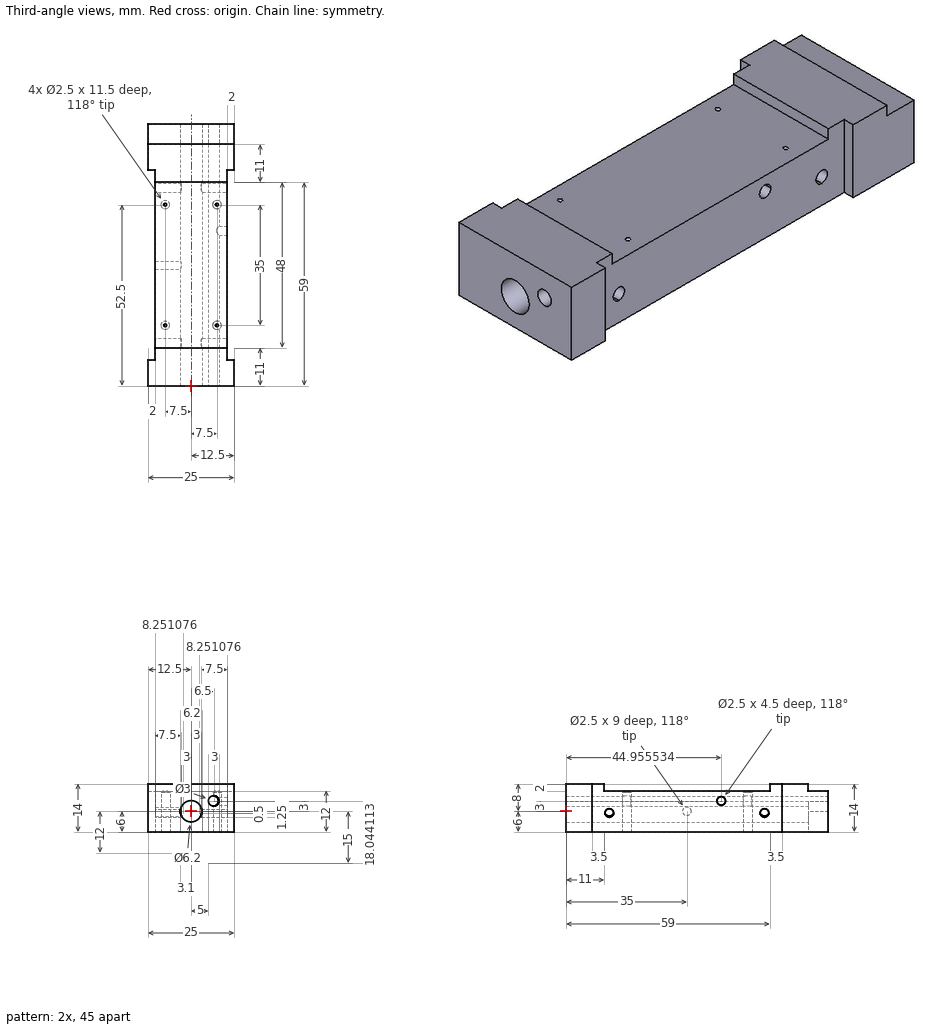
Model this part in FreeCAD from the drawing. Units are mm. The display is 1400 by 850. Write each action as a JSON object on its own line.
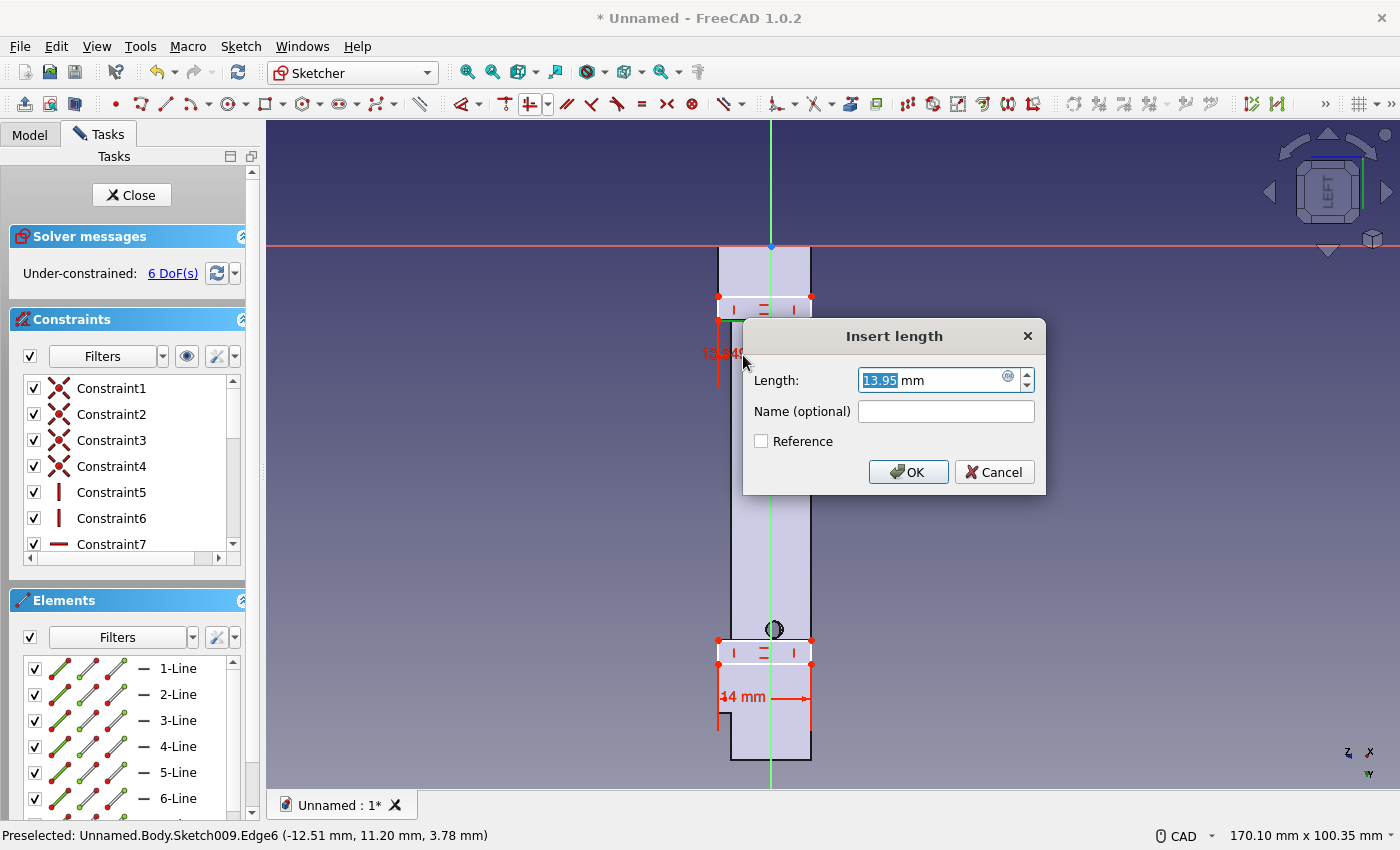
{"action": "type", "text": "14"}
{"action": "key", "text": "Return"}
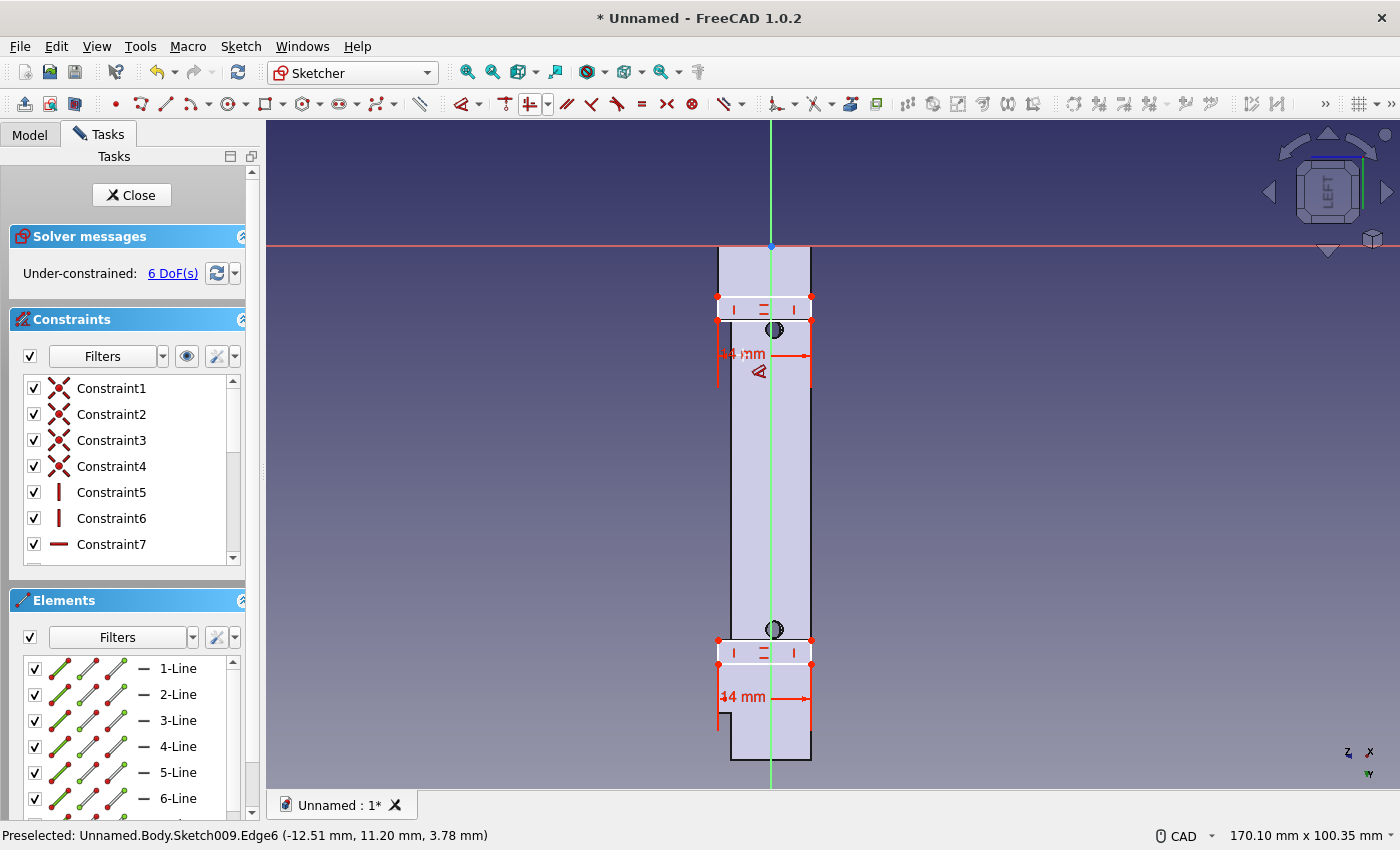
{"action": "left_click", "coordinate": [718, 641]}
{"action": "left_click", "coordinate": [745, 212]}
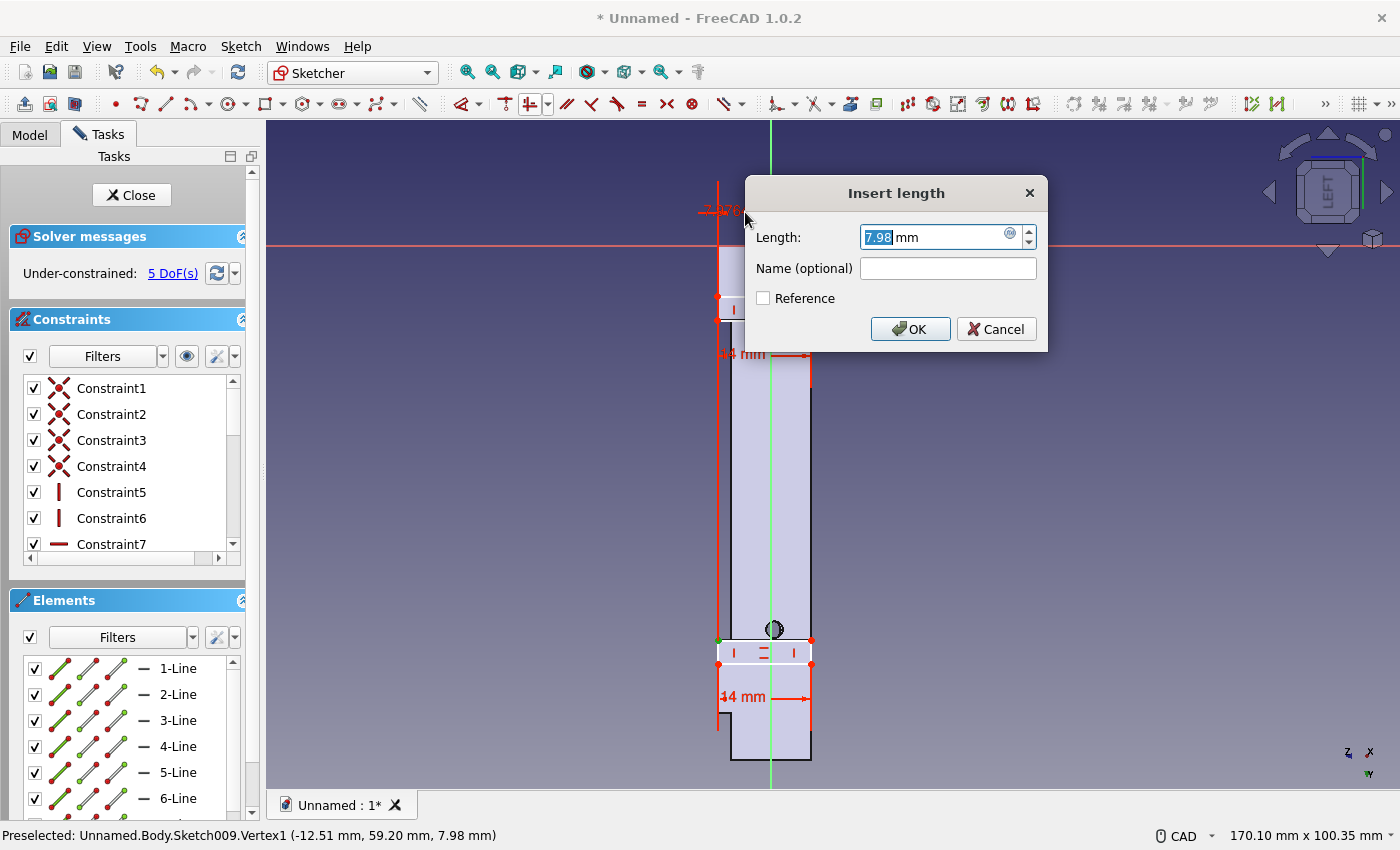
{"action": "type", "text": "8"}
{"action": "key", "text": "Return"}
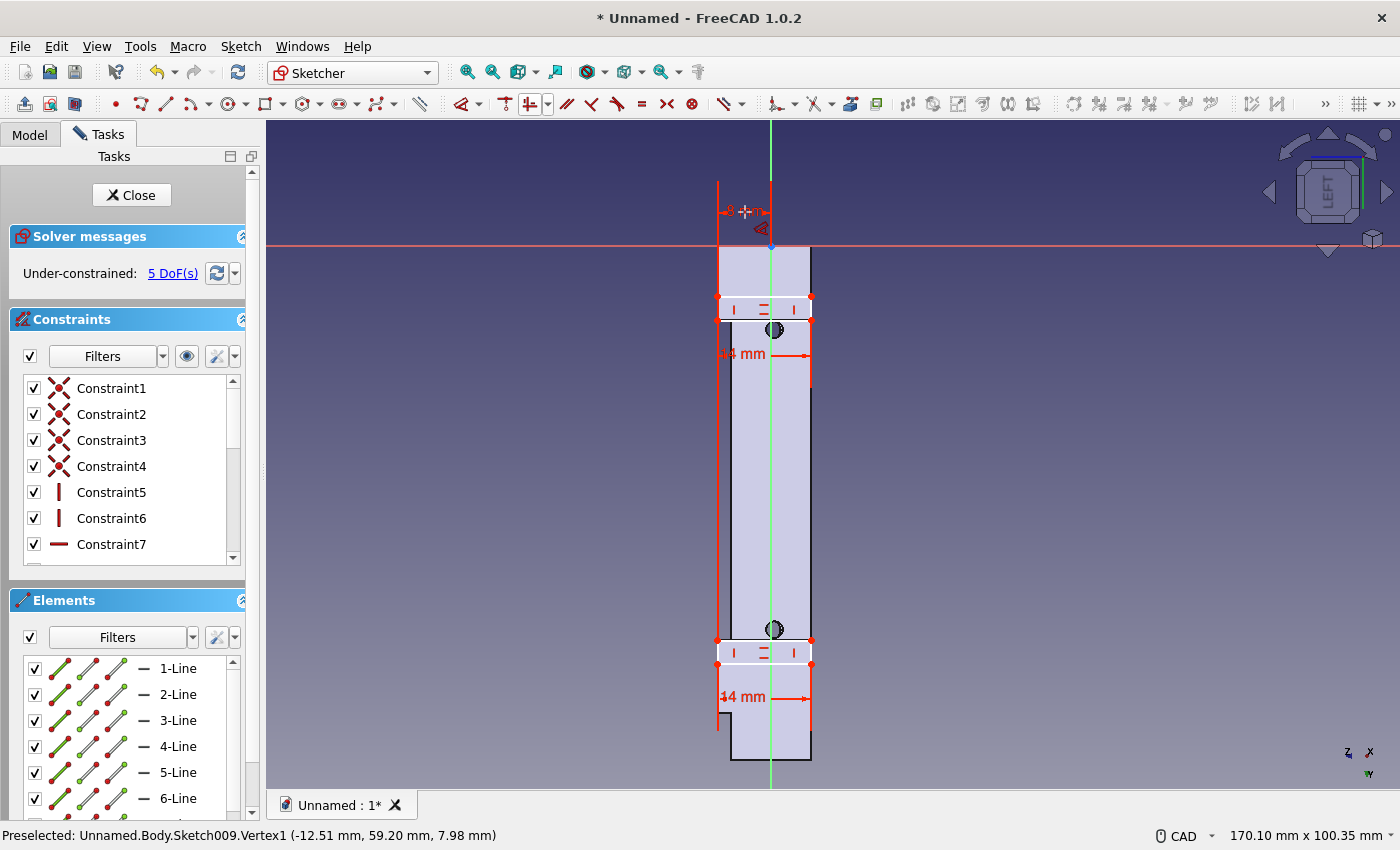
{"action": "left_click", "coordinate": [718, 297]}
{"action": "left_click", "coordinate": [744, 188]}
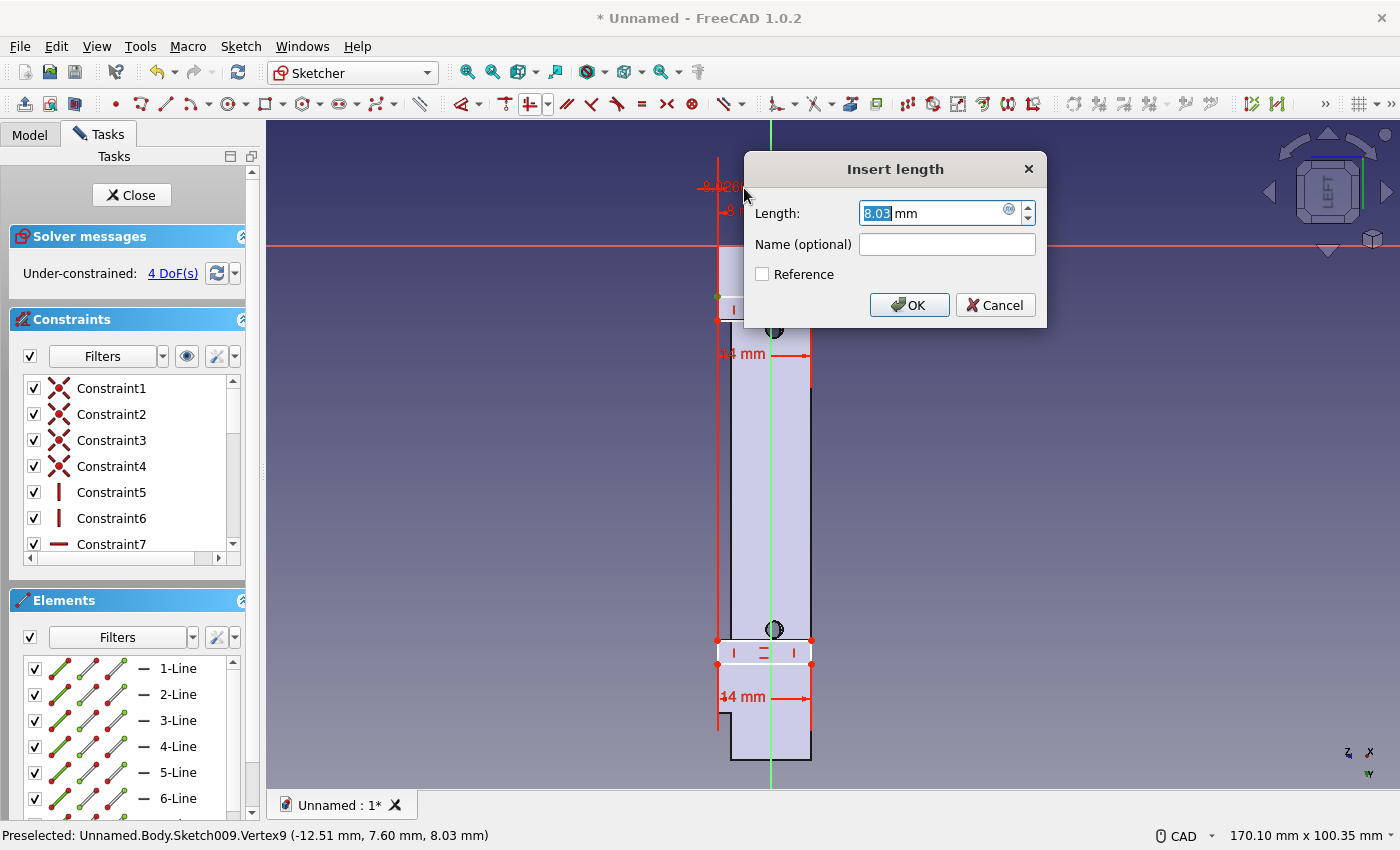
{"action": "type", "text": "8"}
{"action": "key", "text": "Return"}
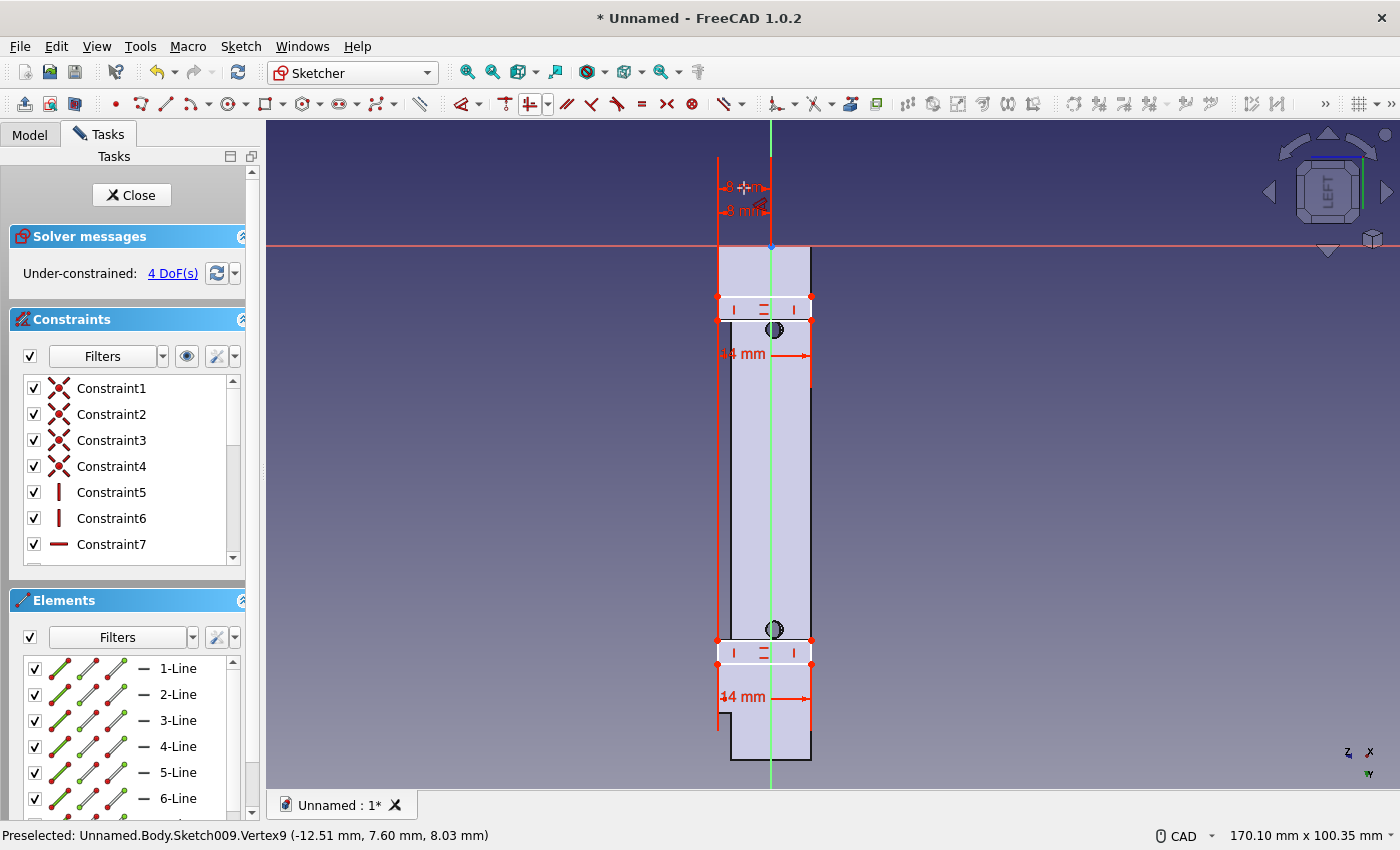
{"action": "scroll", "coordinate": [718, 650], "scroll_direction": "up", "scroll_amount": 3}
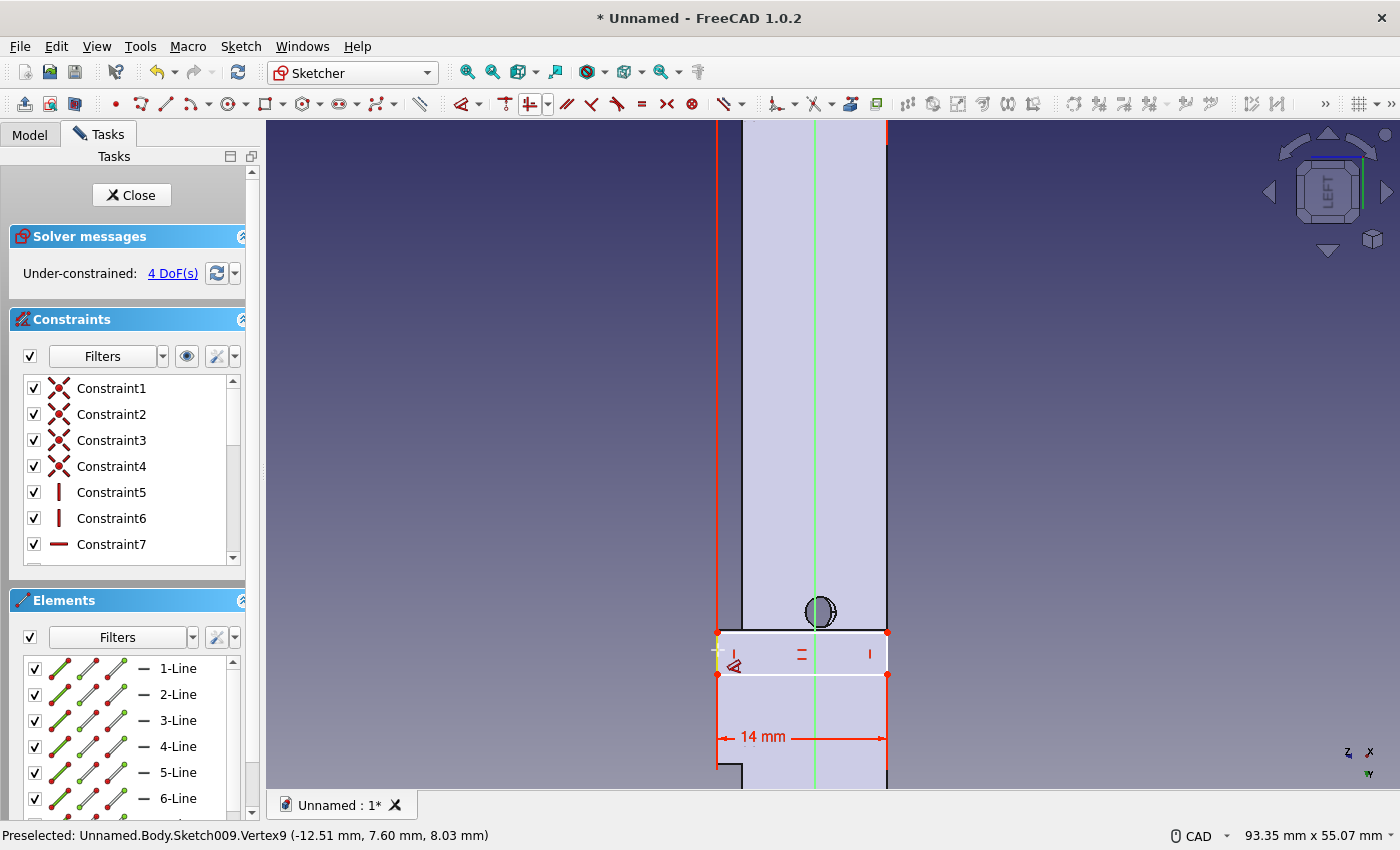
{"action": "left_click", "coordinate": [717, 650]}
{"action": "left_click", "coordinate": [683, 654]}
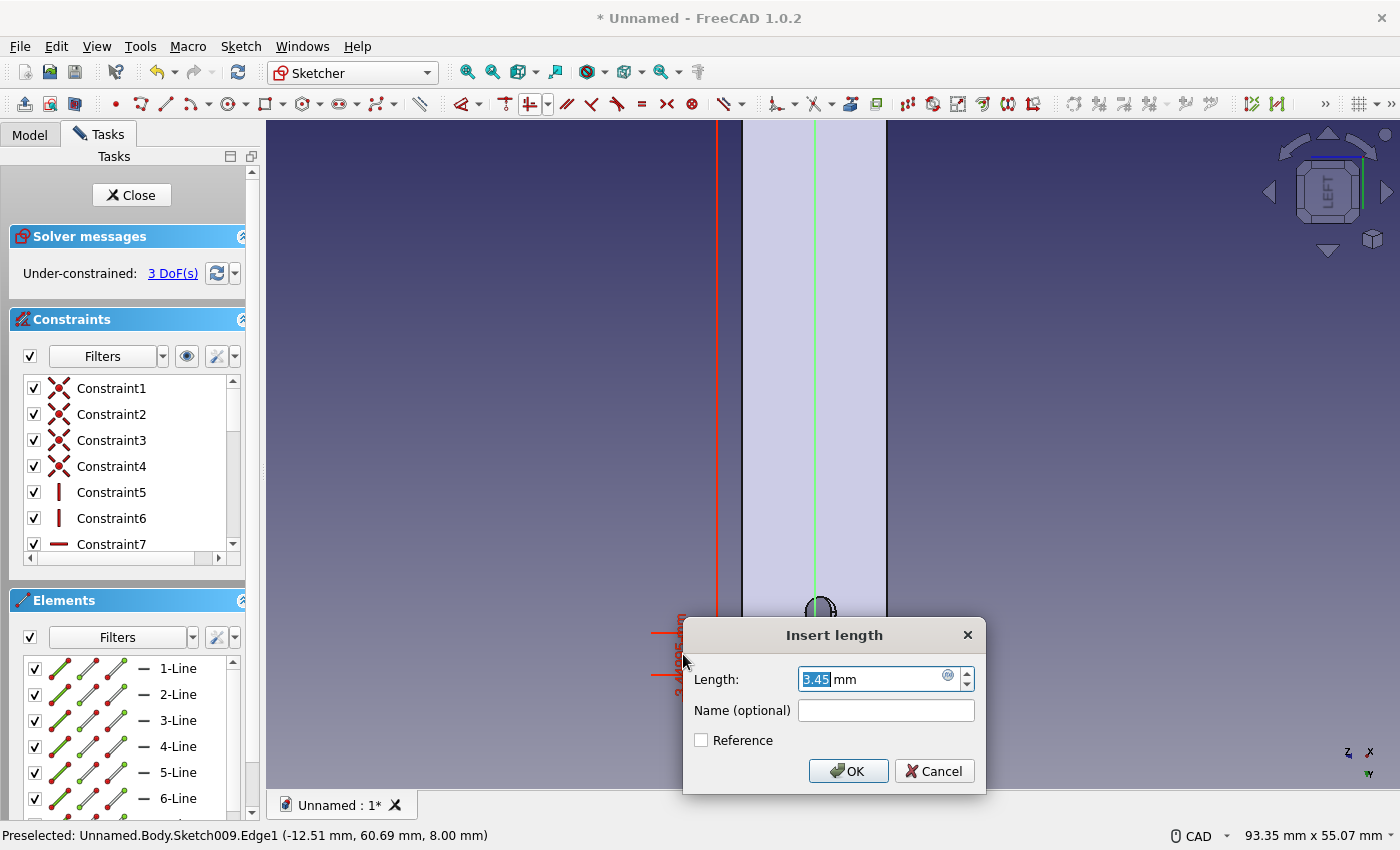
{"action": "type", "text": "3.5"}
{"action": "key", "text": "Return"}